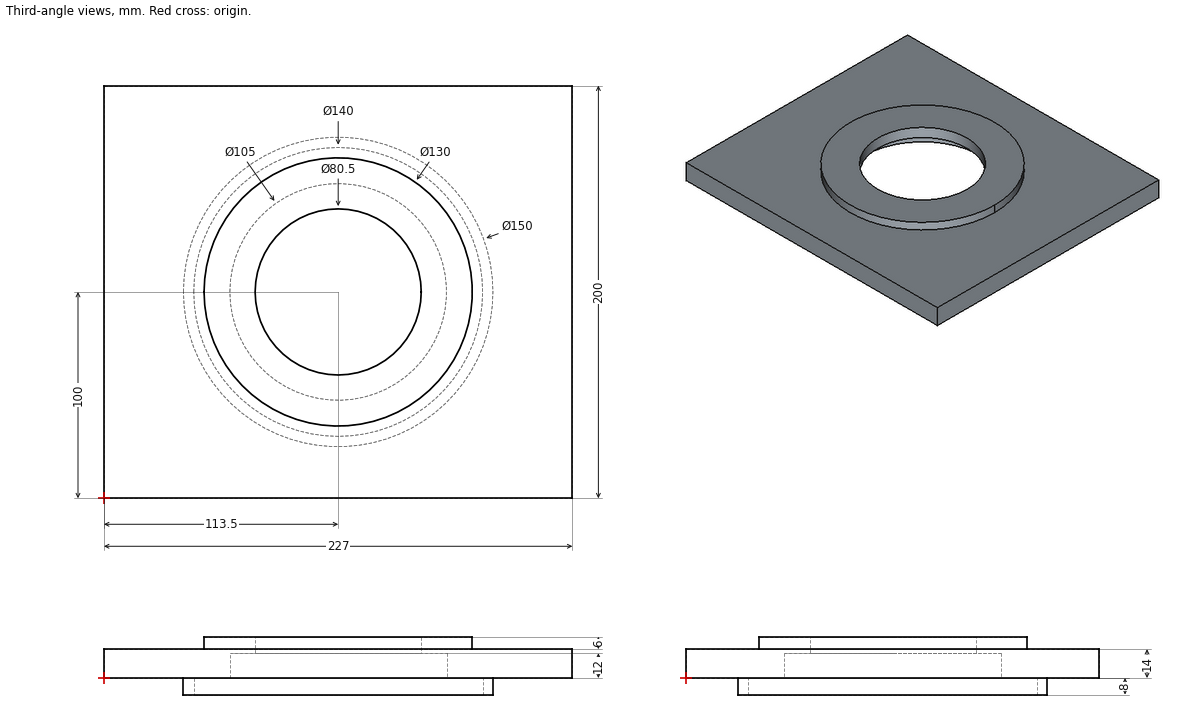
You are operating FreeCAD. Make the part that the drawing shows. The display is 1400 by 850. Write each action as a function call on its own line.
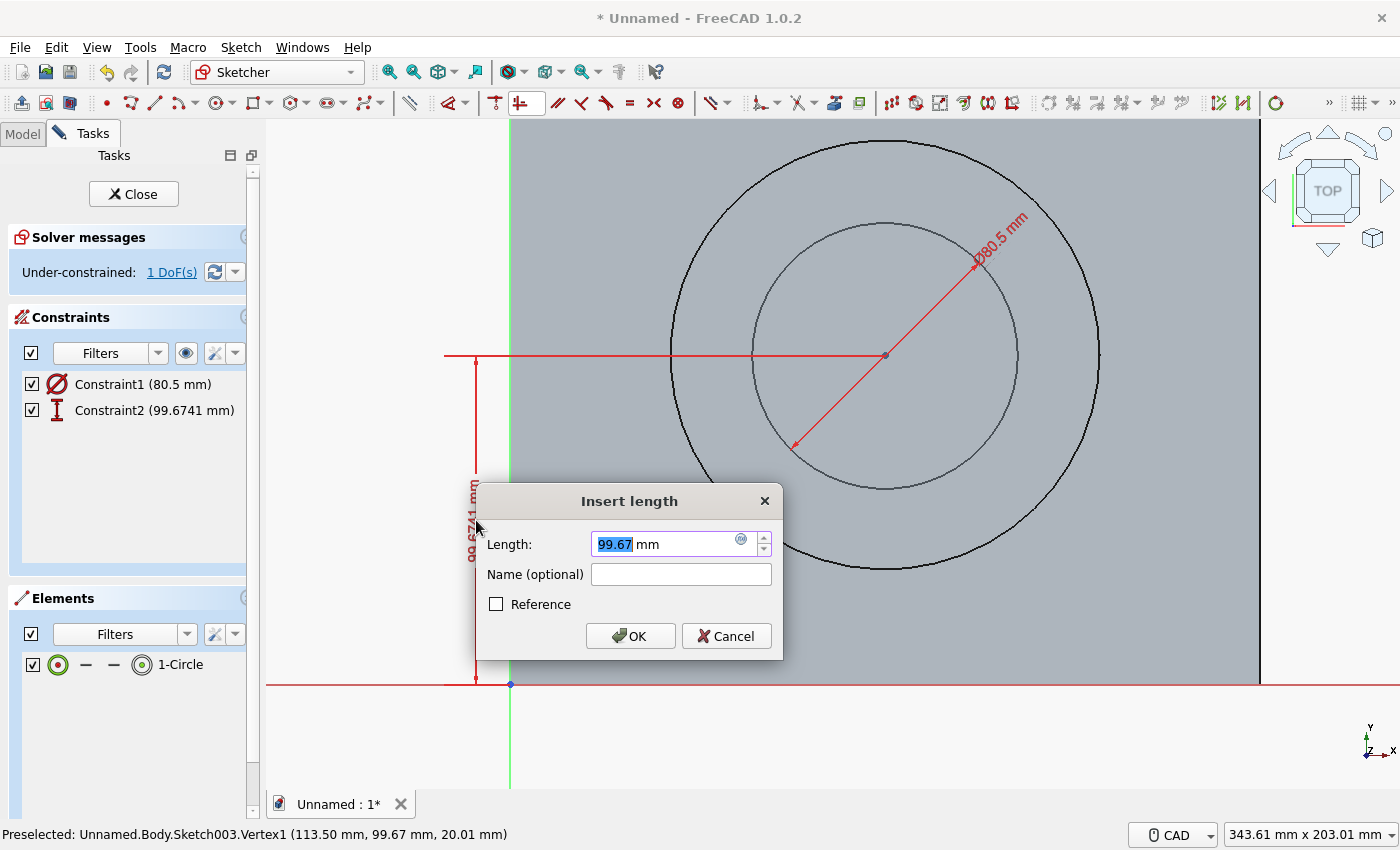
text(100)
key(Return)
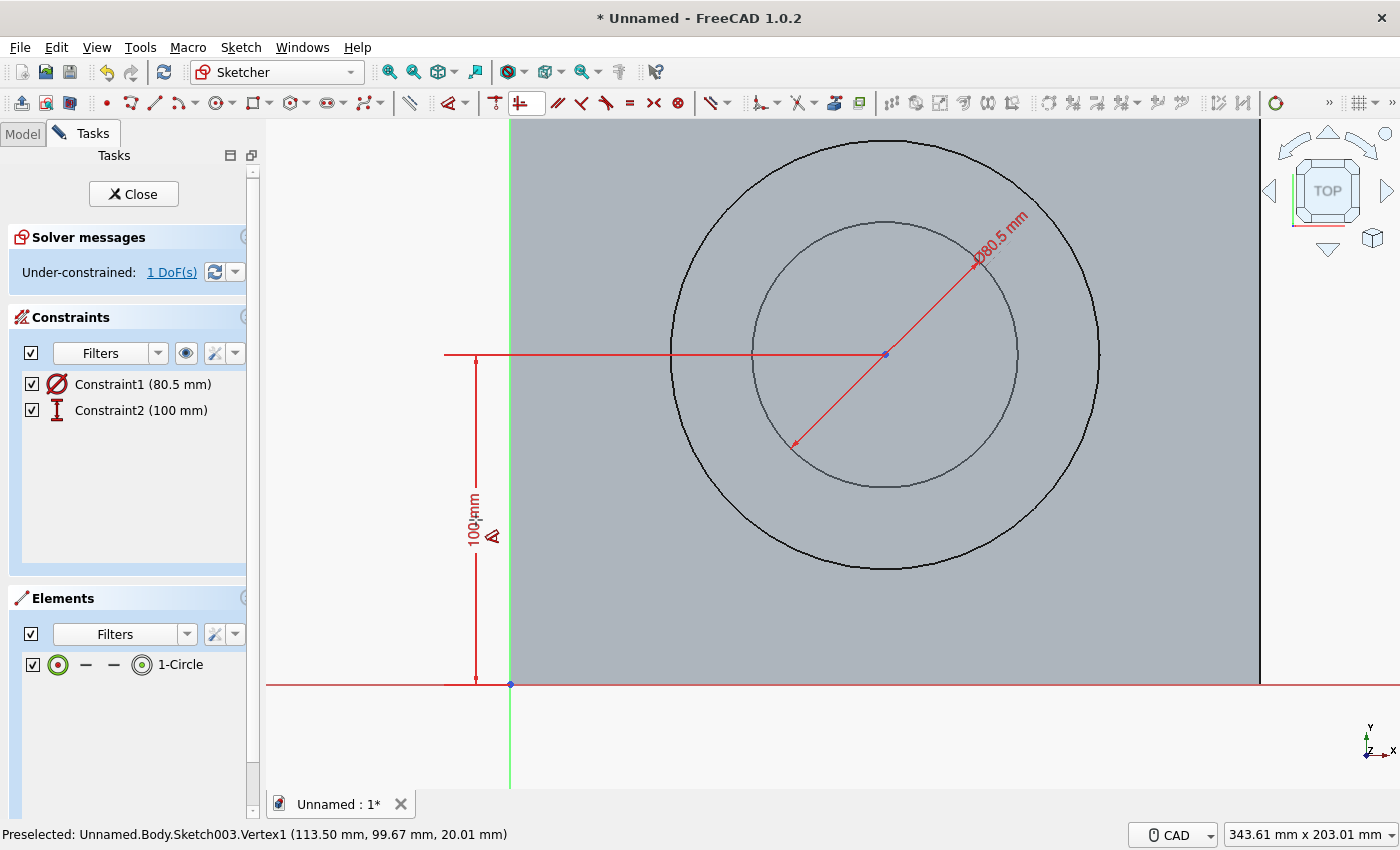
click(885, 355)
click(698, 719)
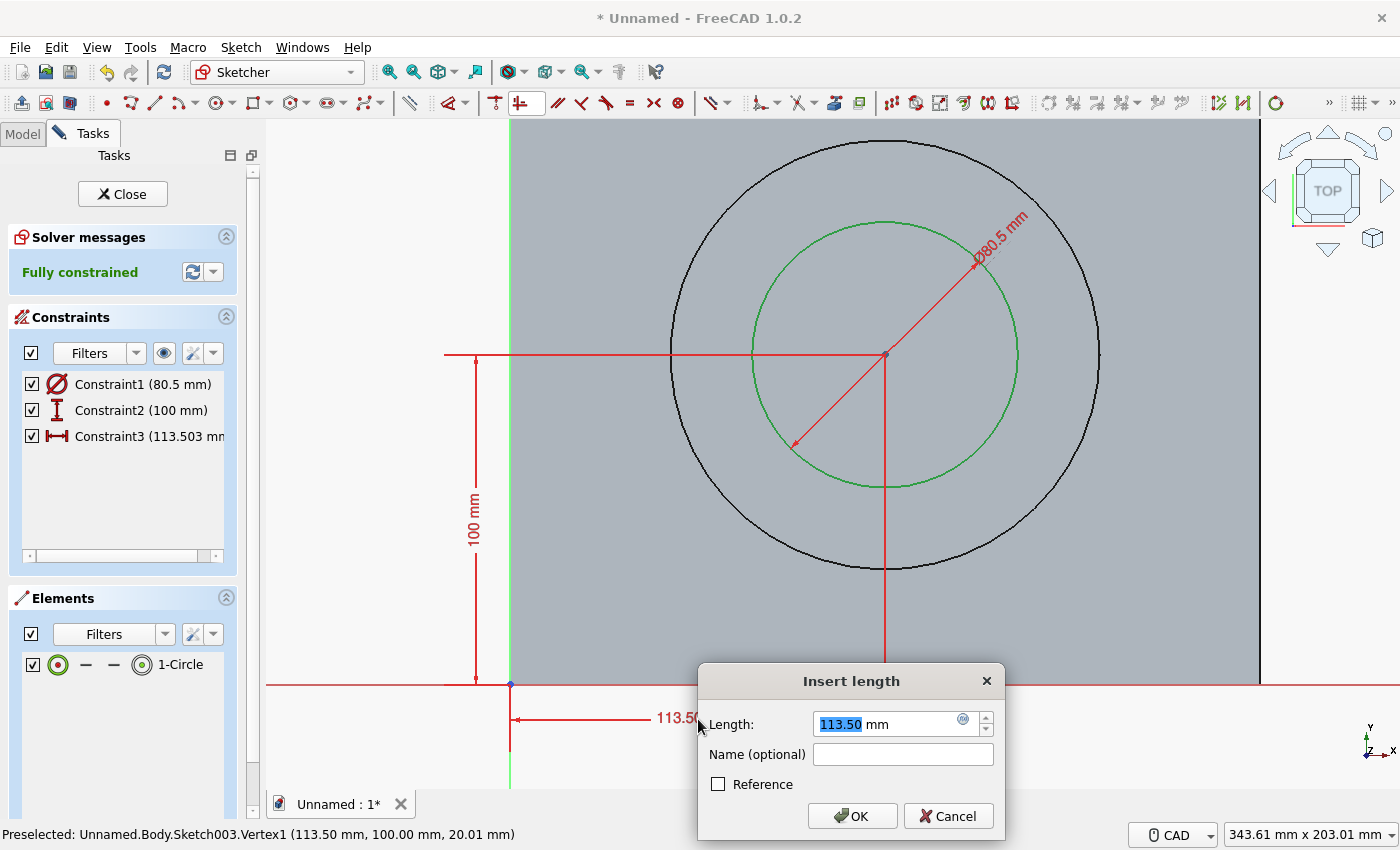
text(113.5)
key(Return)
key(Escape)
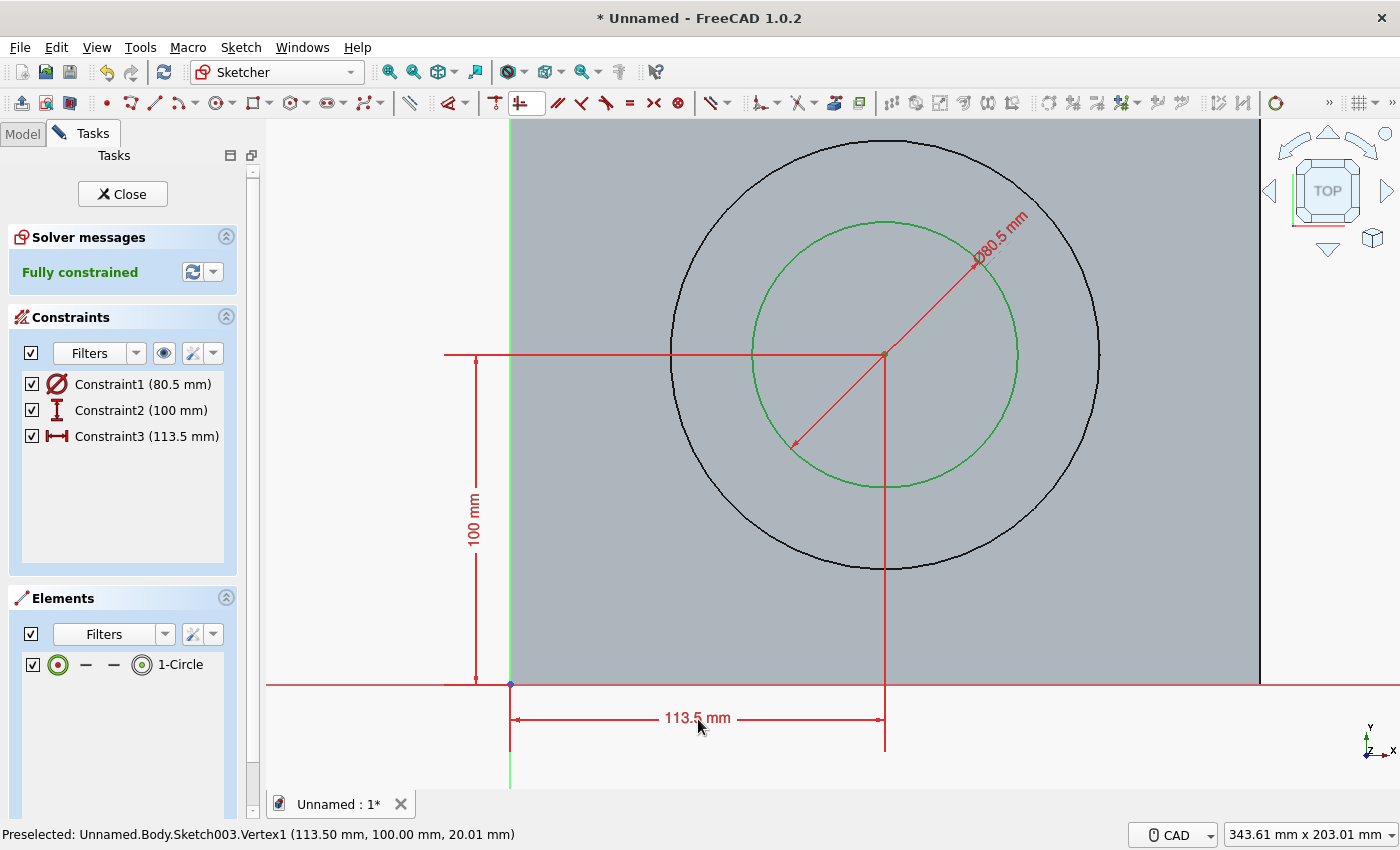
click(123, 194)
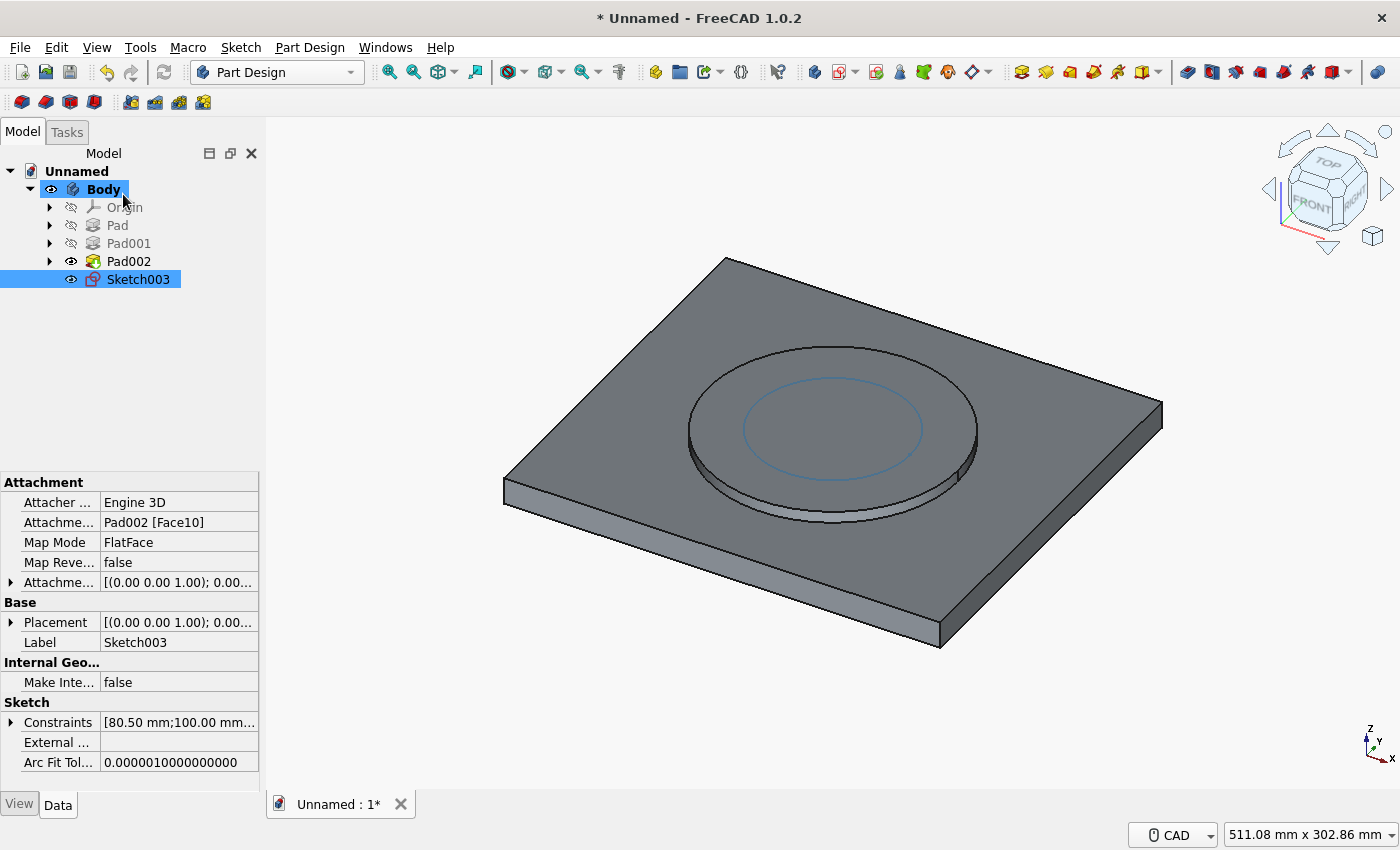
click(1188, 72)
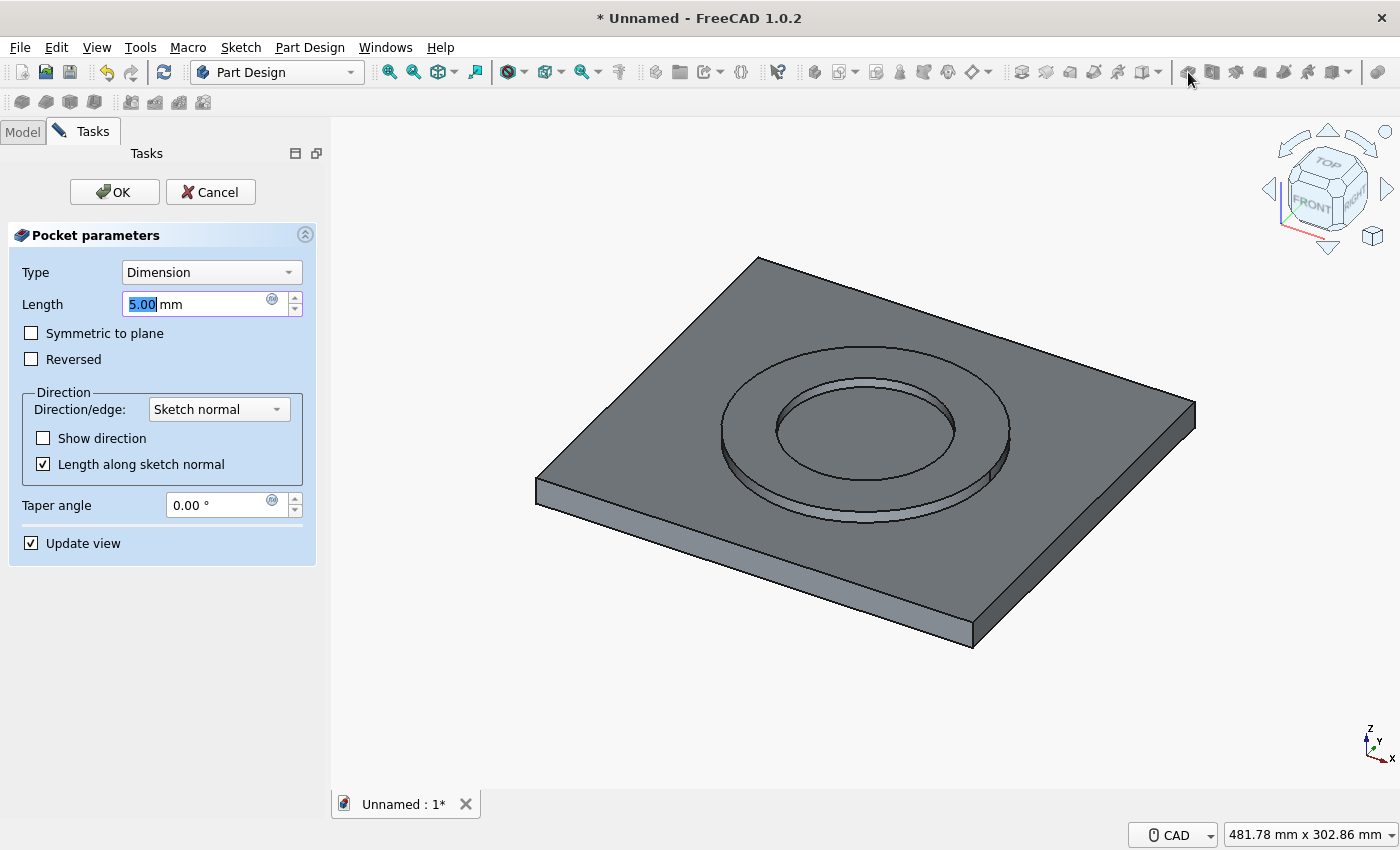
click(212, 272)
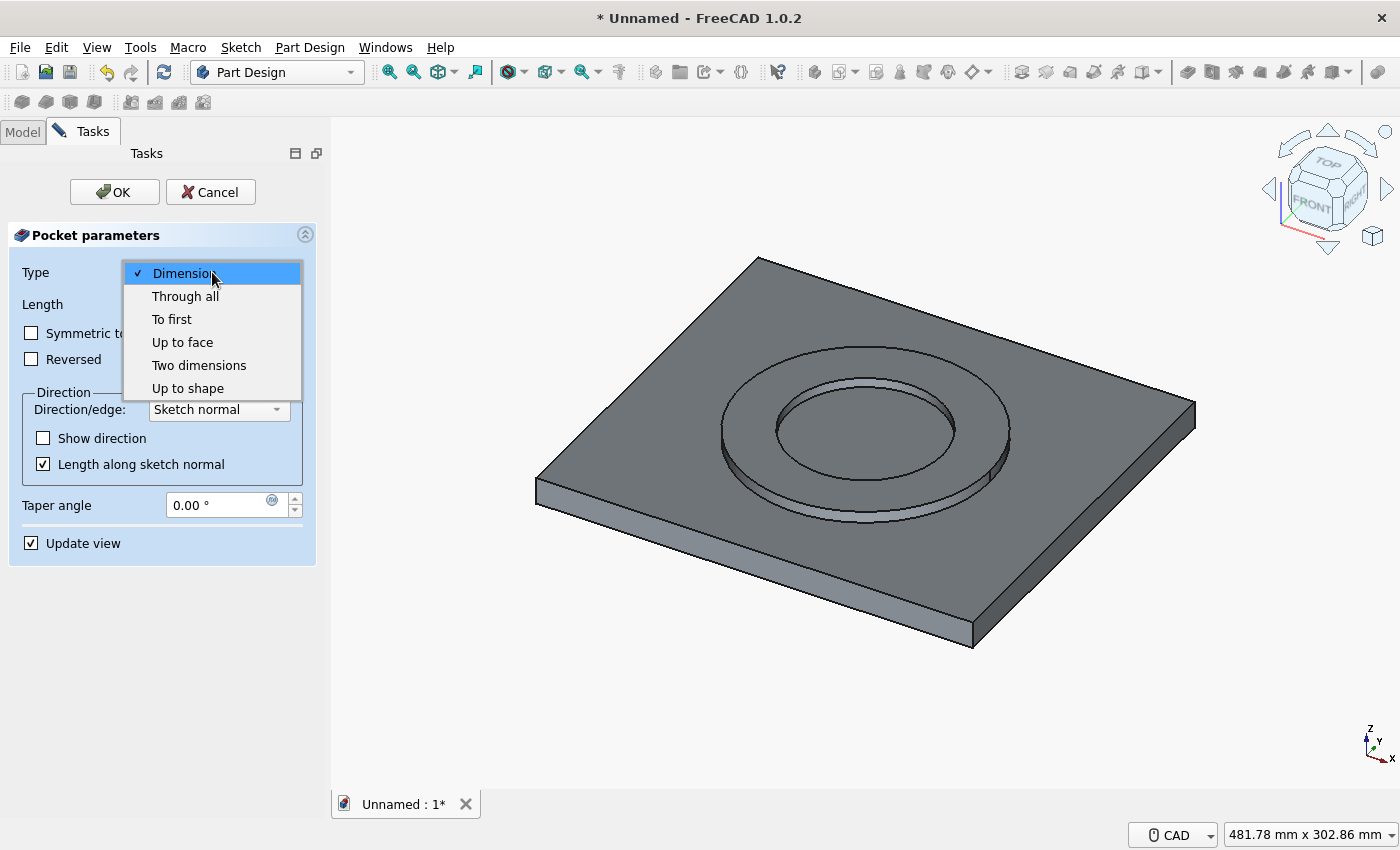
click(212, 296)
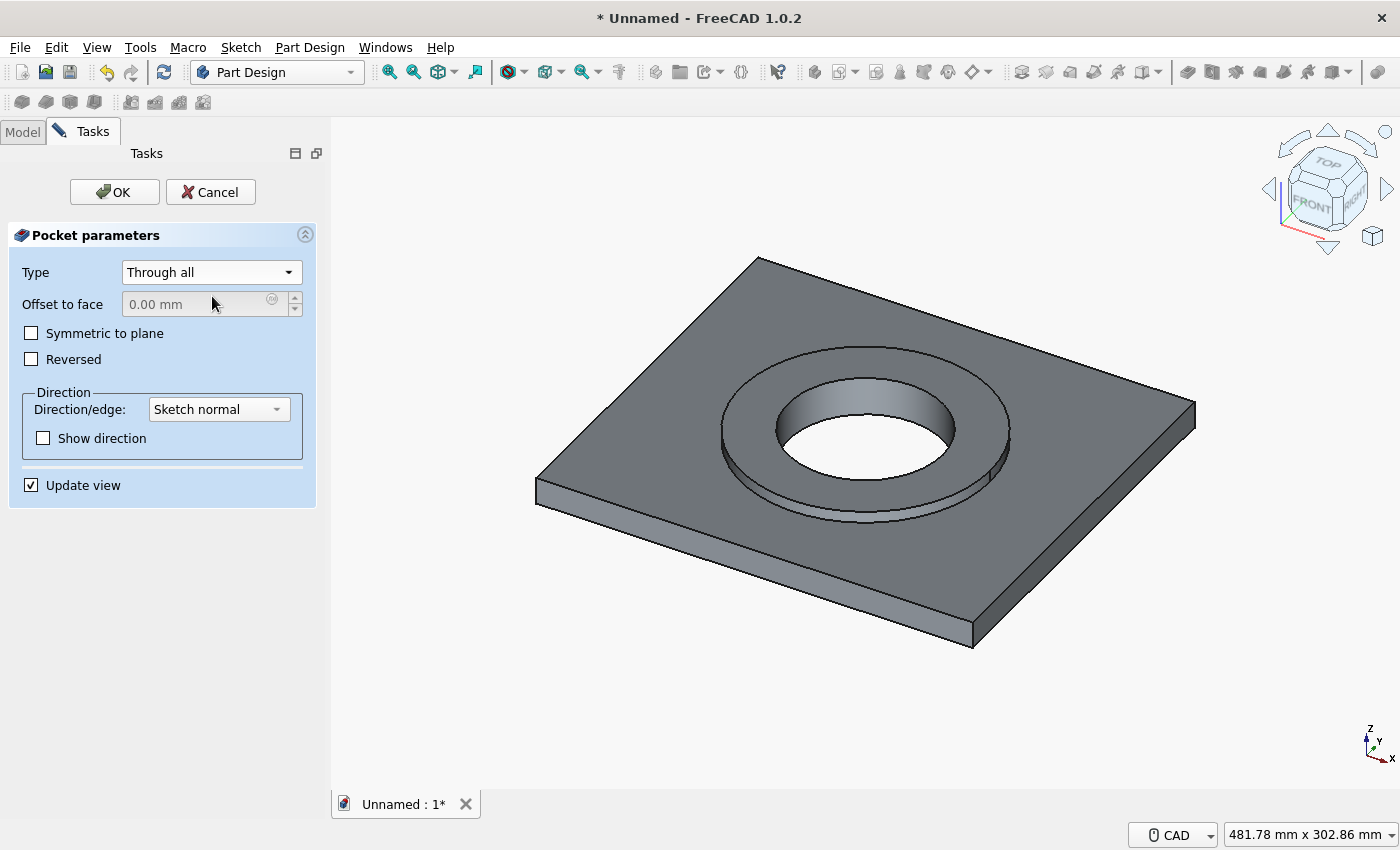
click(115, 192)